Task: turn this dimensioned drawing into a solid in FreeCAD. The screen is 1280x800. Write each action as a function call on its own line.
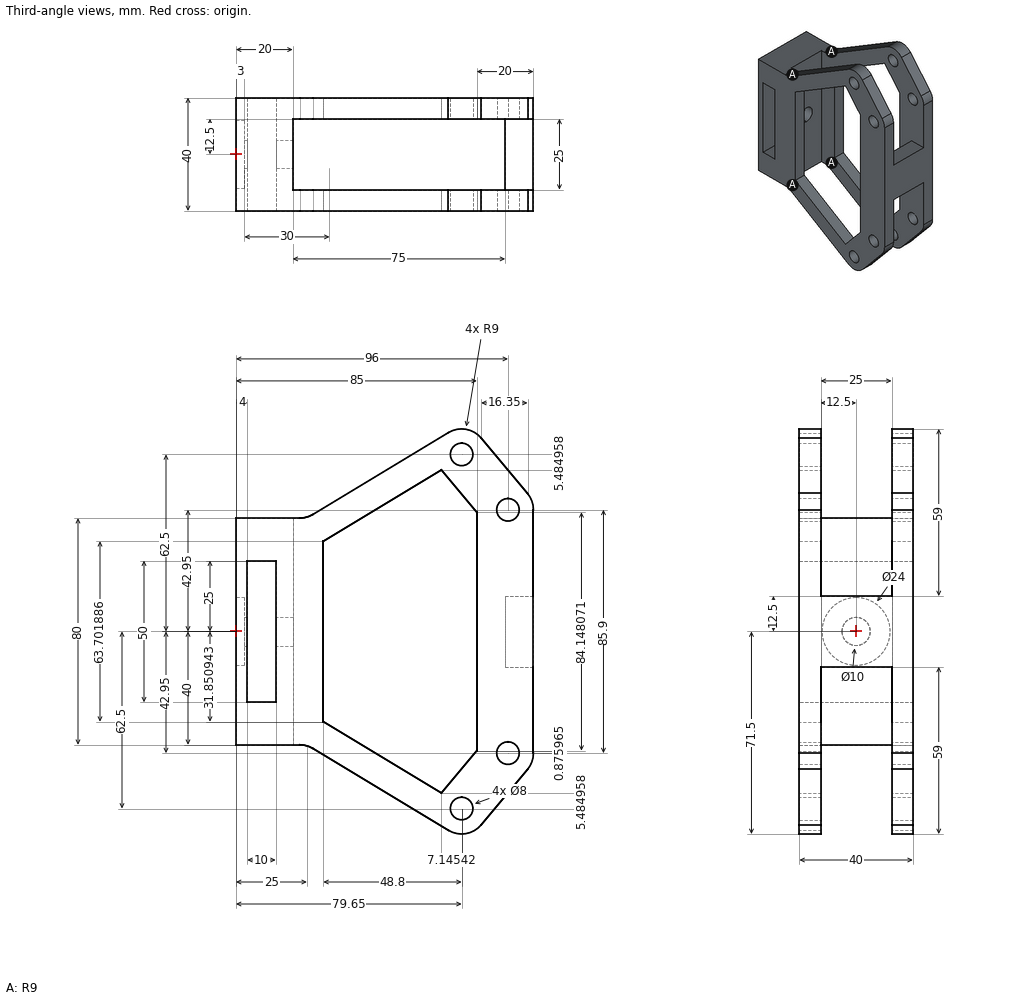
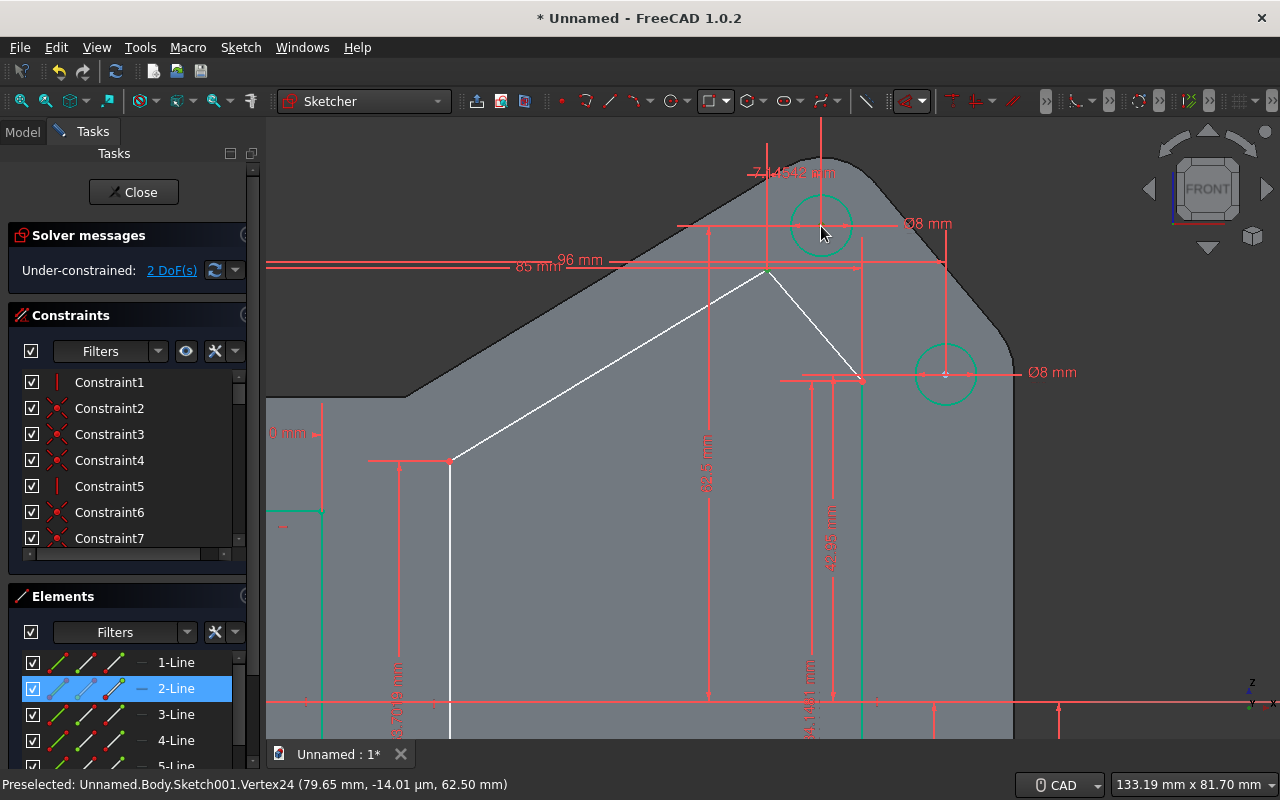
key(i)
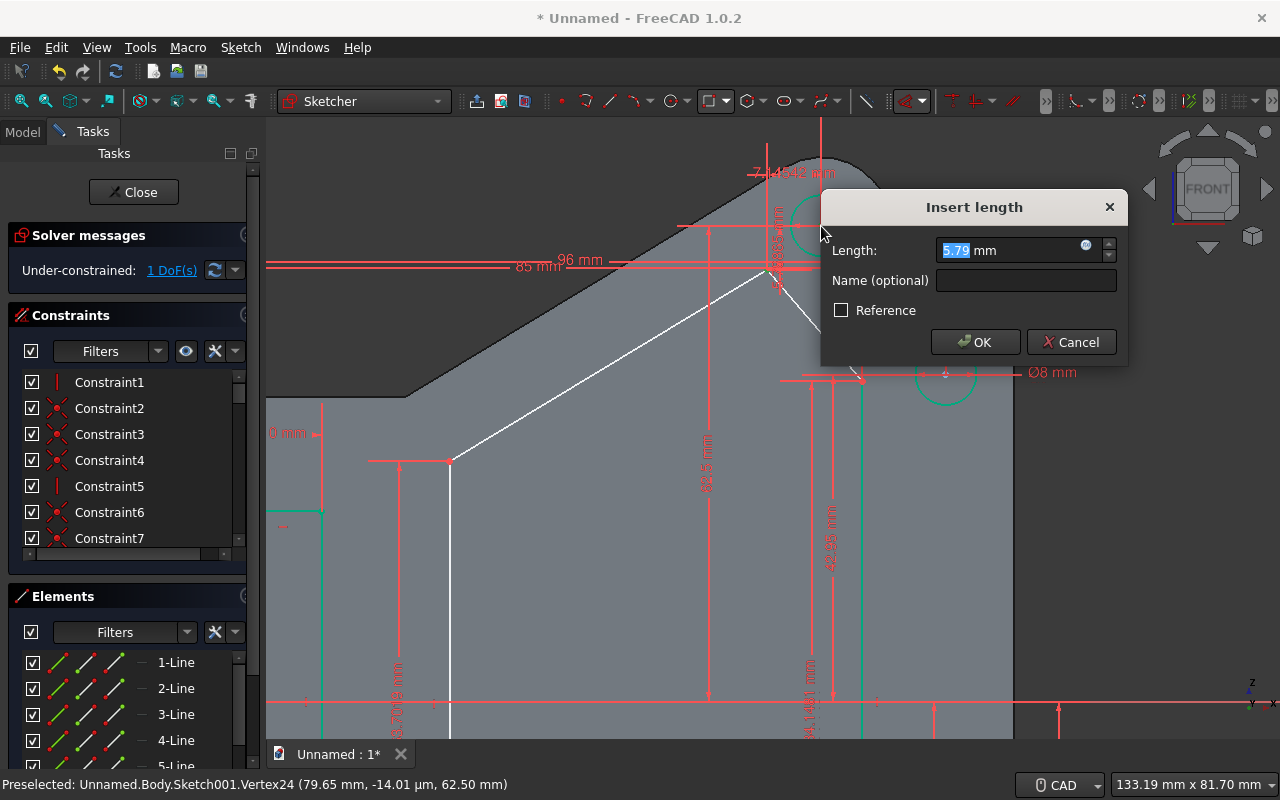
text(5.484958)
key(Return)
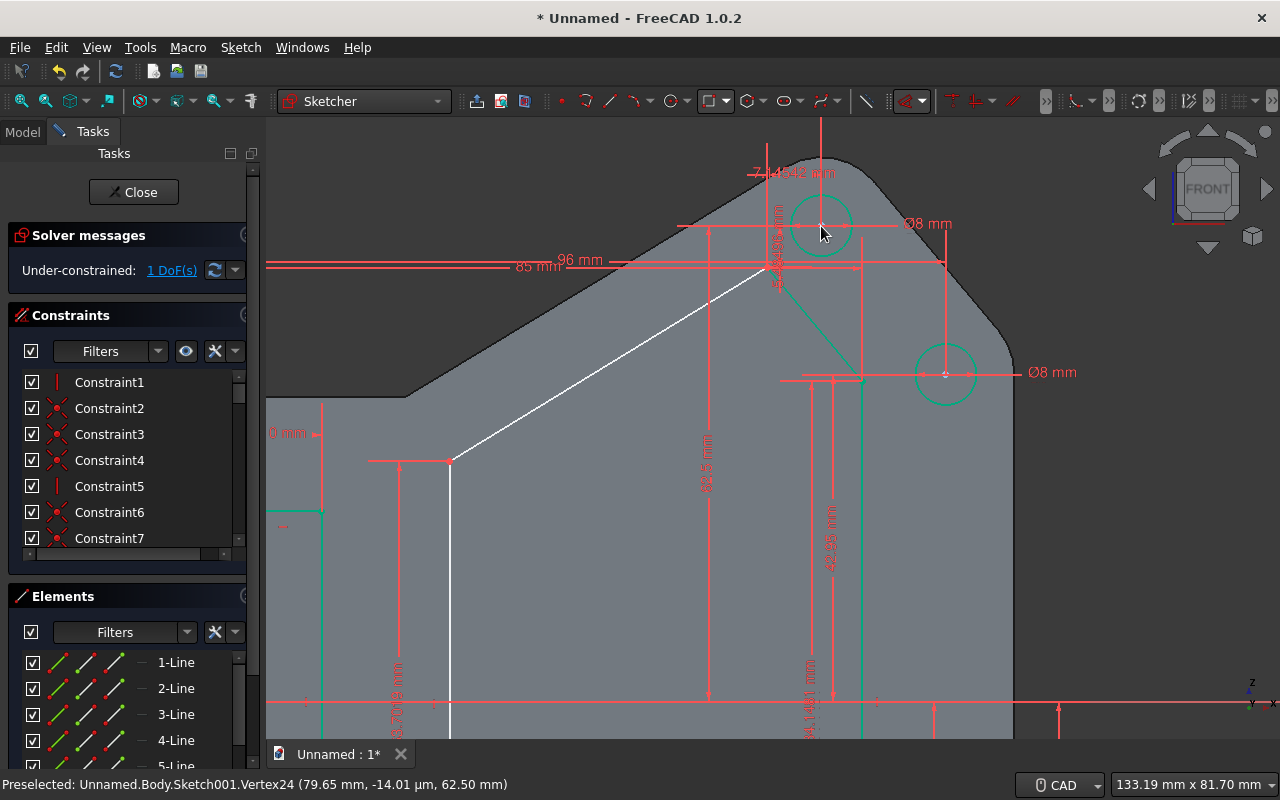
scroll(768, 269, down, 5)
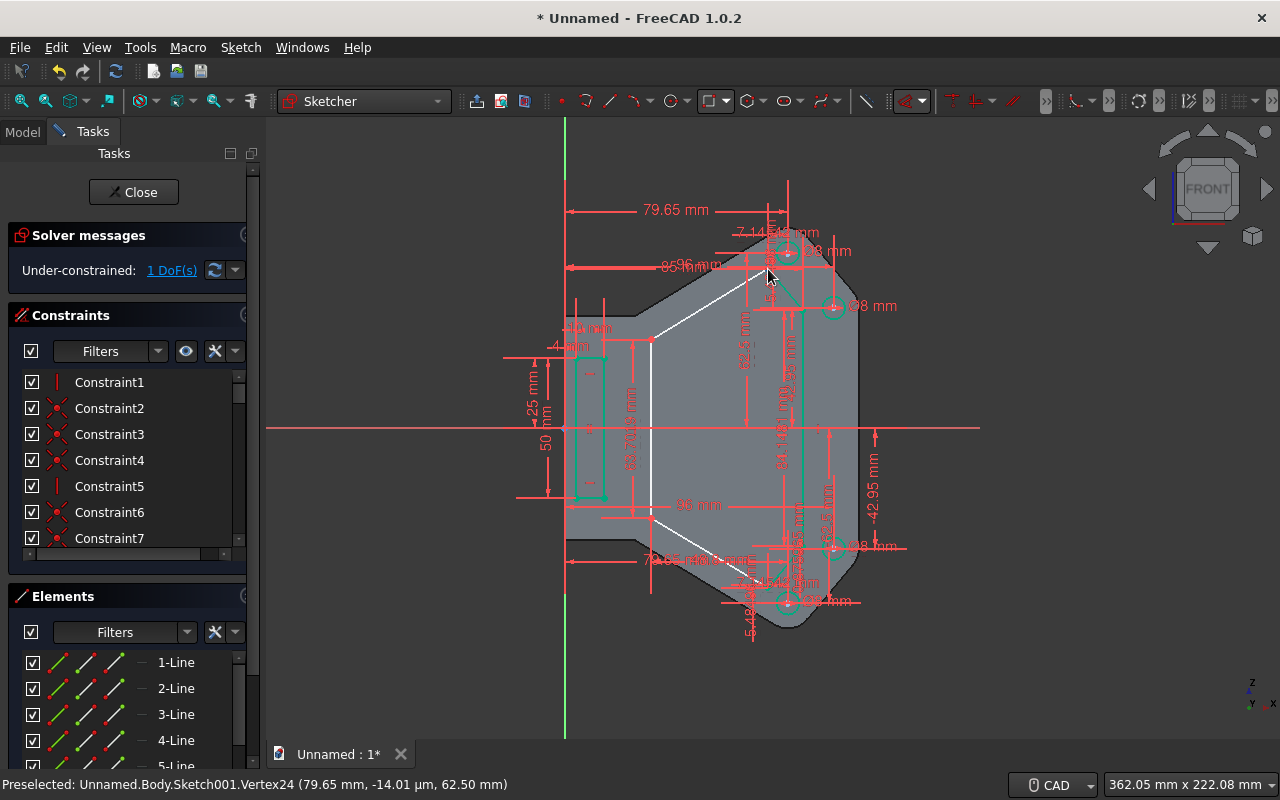
click(651, 518)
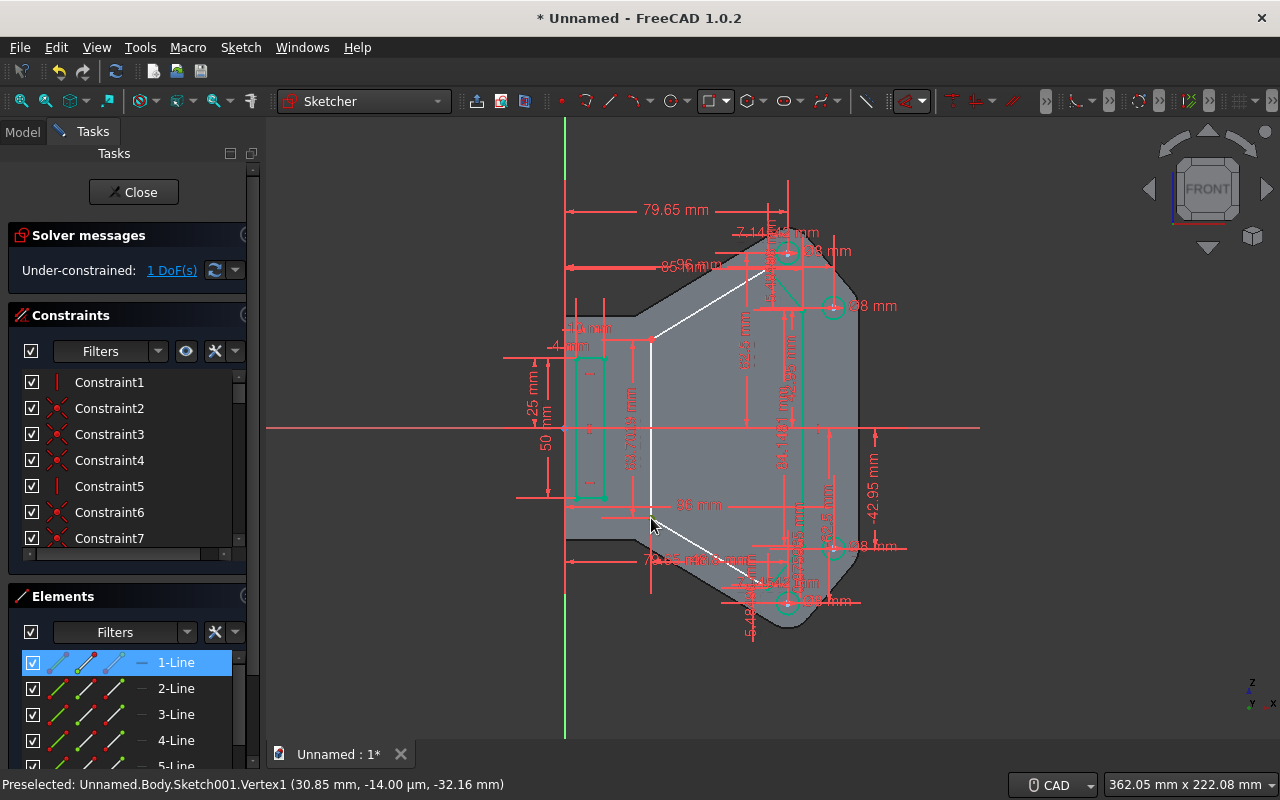
key(i)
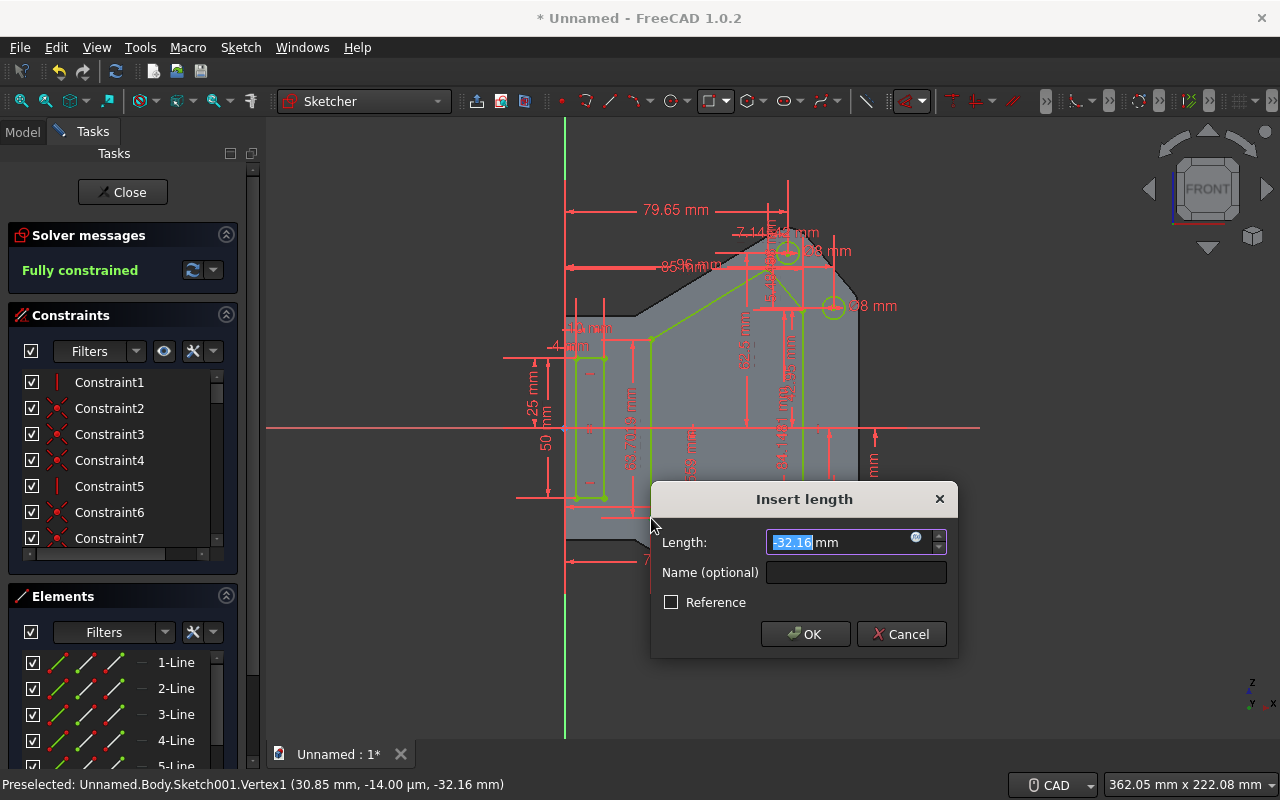
text(-31.850943)
key(Return)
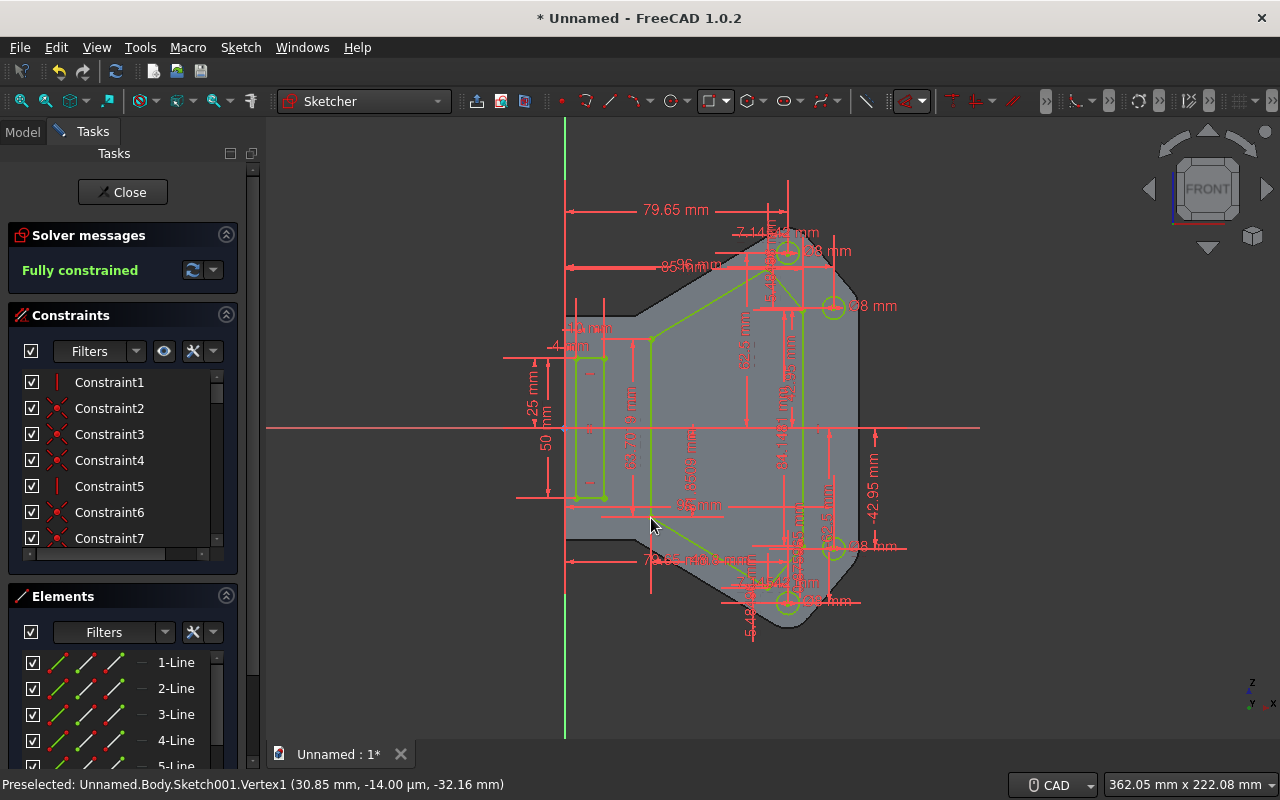
click(123, 192)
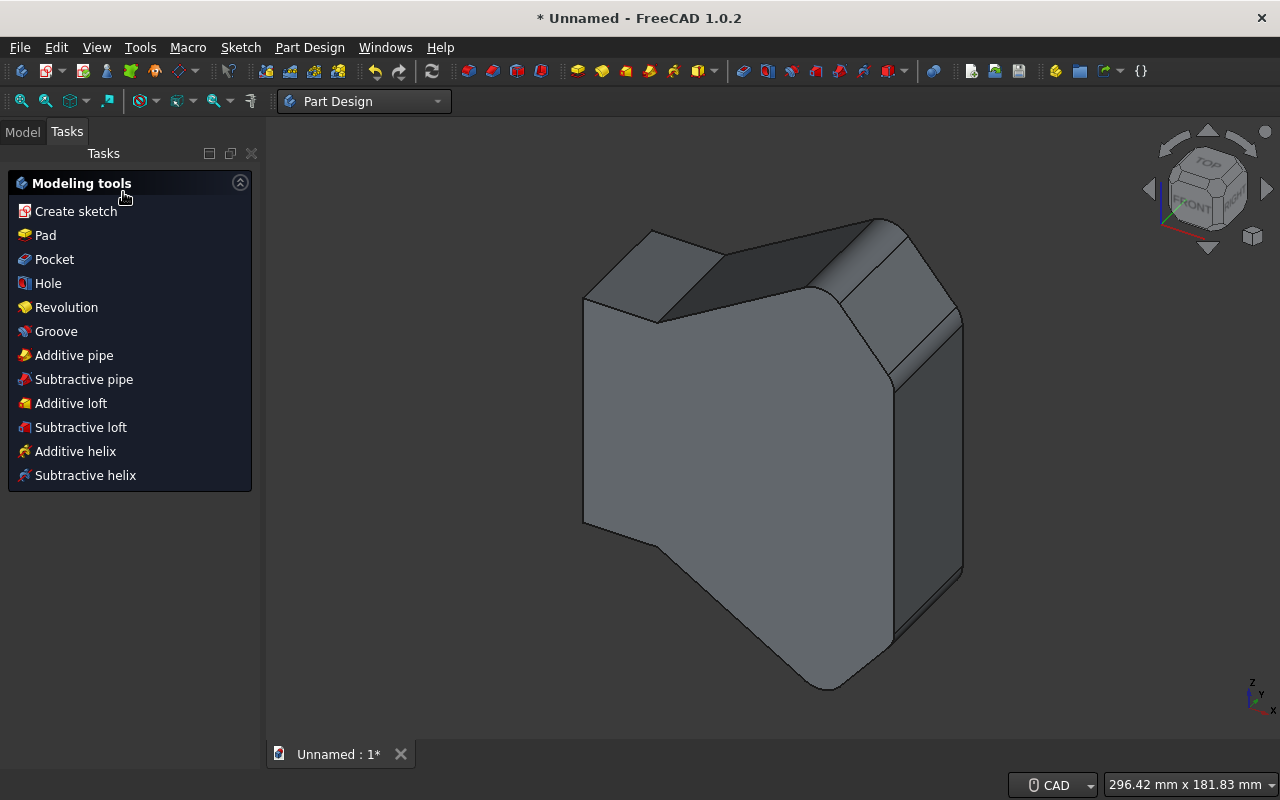
click(744, 72)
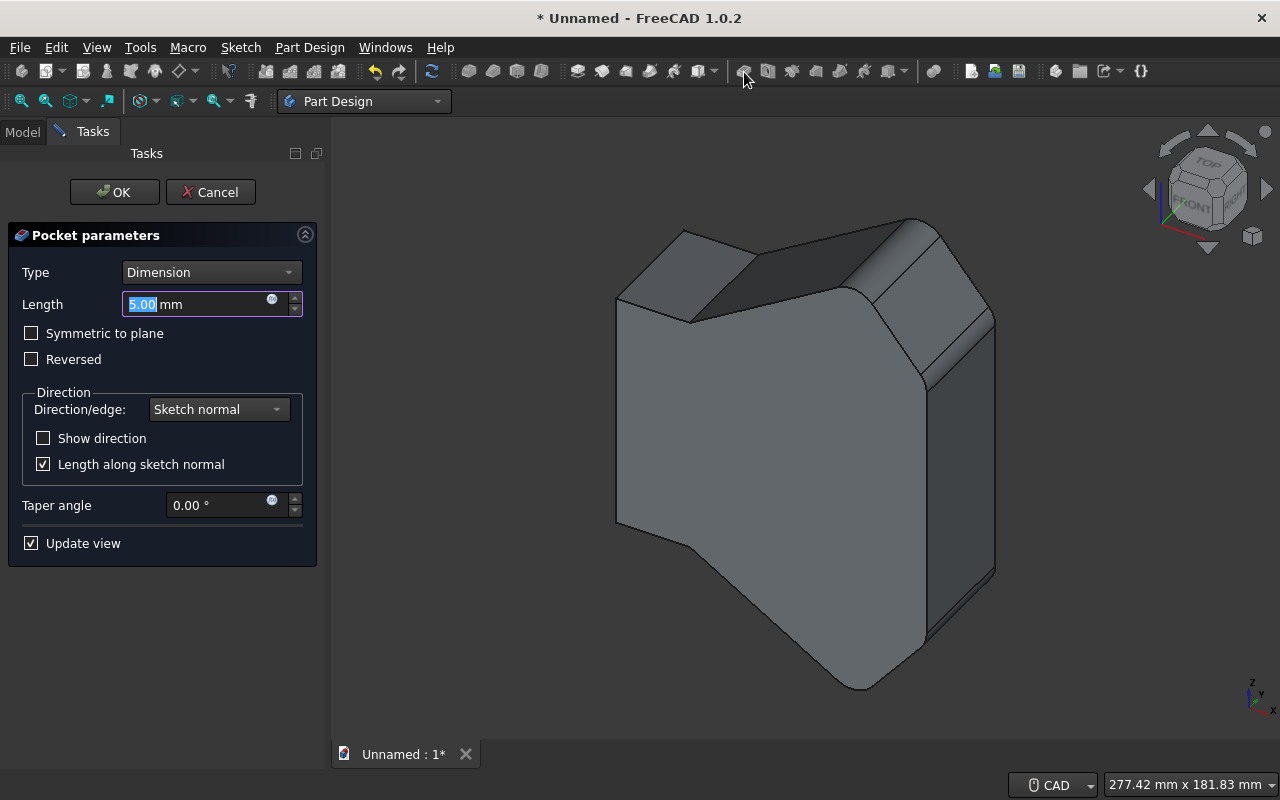
text(40)
key(Tab)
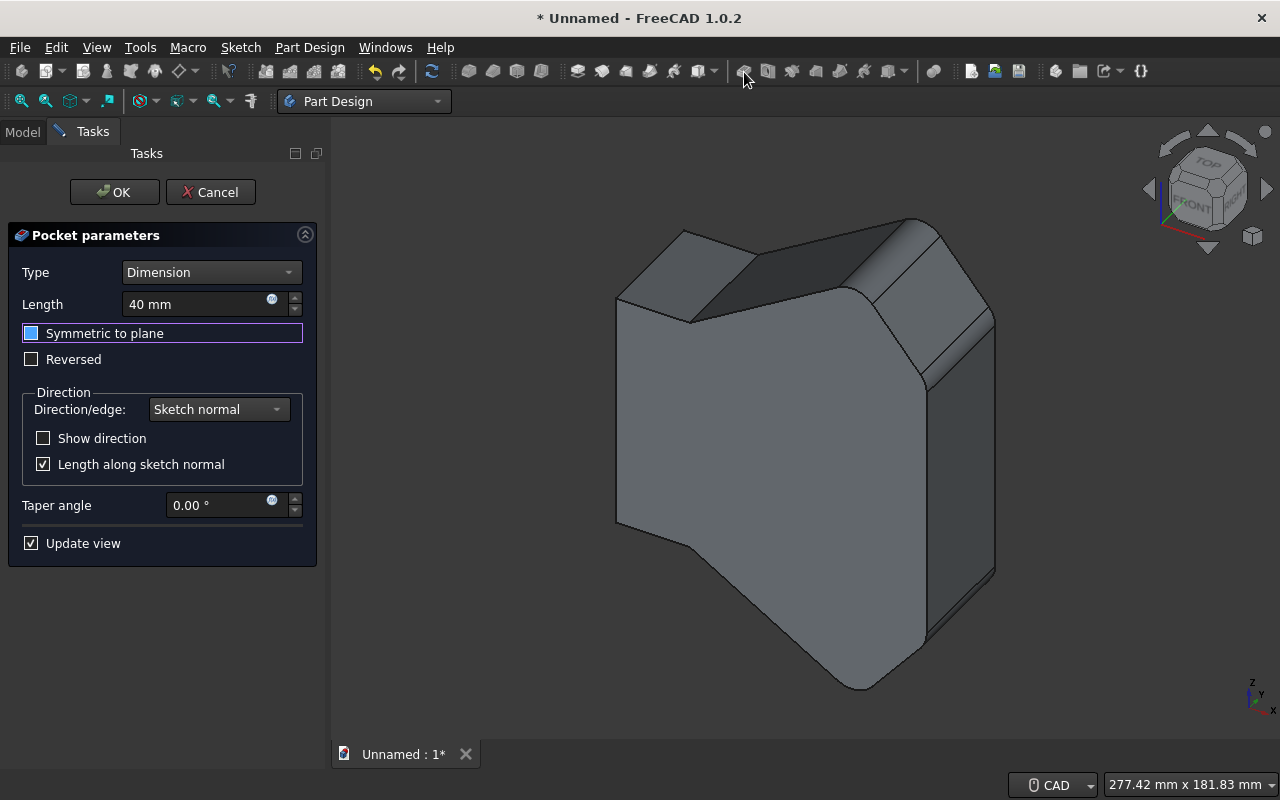
click(30, 333)